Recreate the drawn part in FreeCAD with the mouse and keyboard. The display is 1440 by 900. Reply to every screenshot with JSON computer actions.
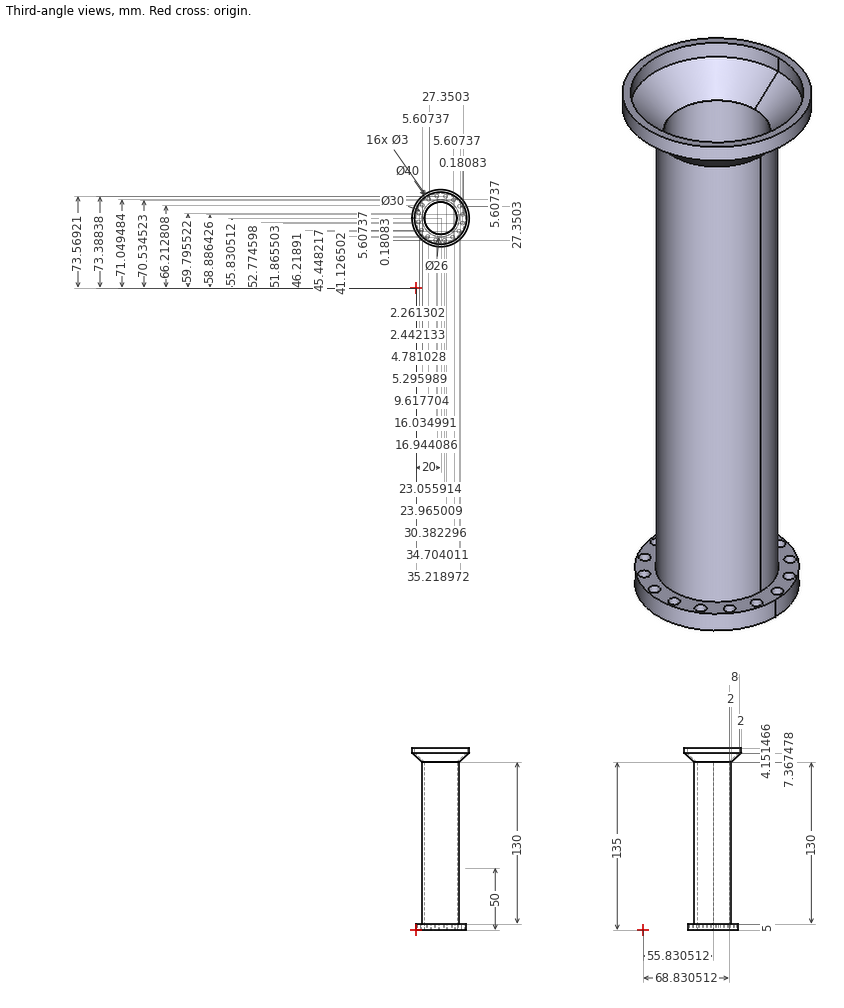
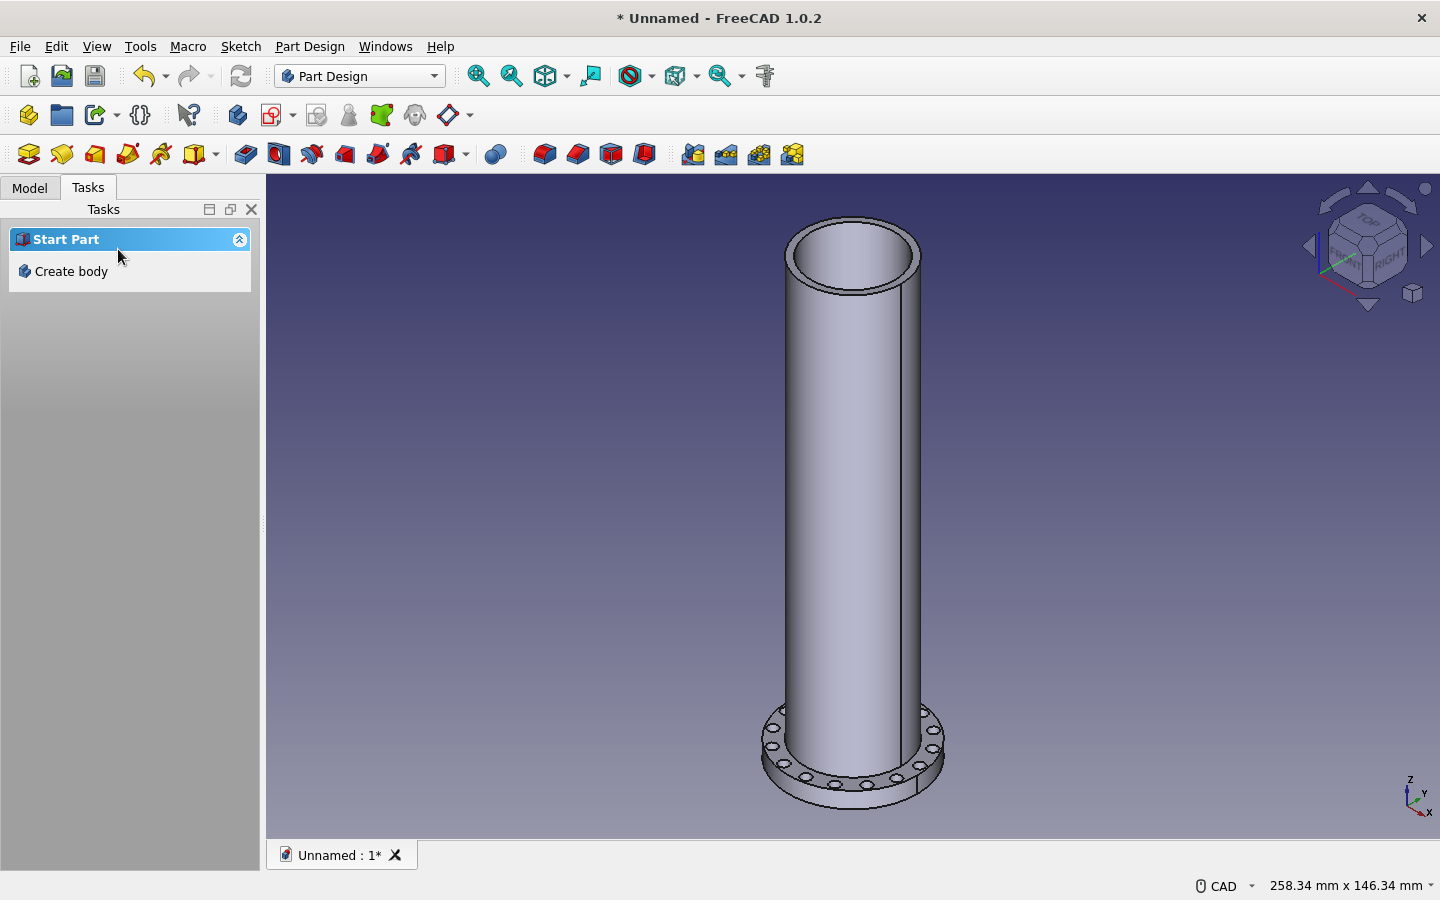
{"action": "left_click", "coordinate": [238, 116]}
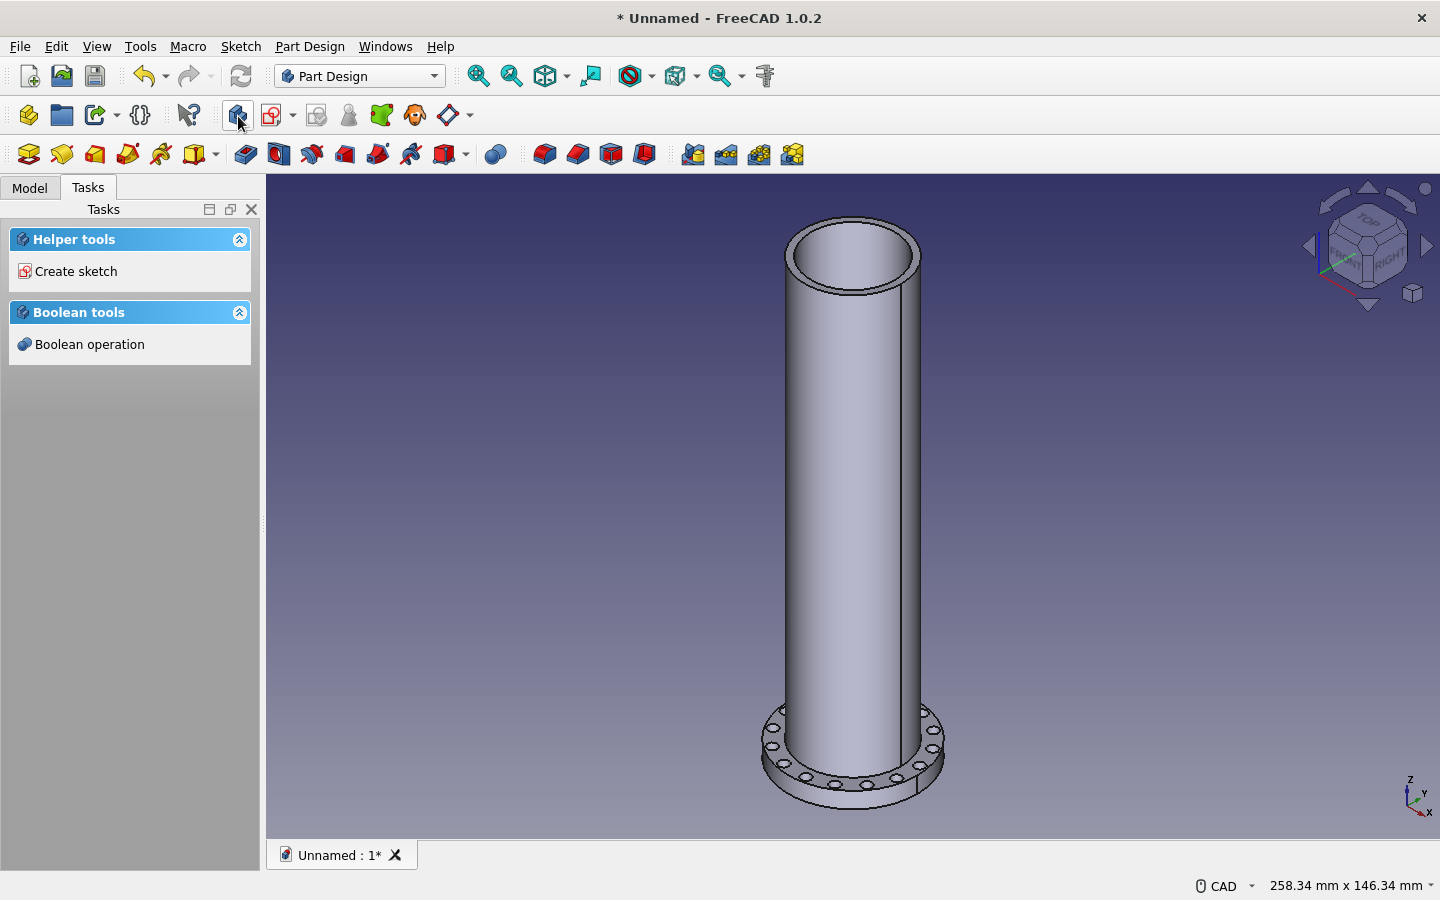
{"action": "left_click", "coordinate": [30, 188]}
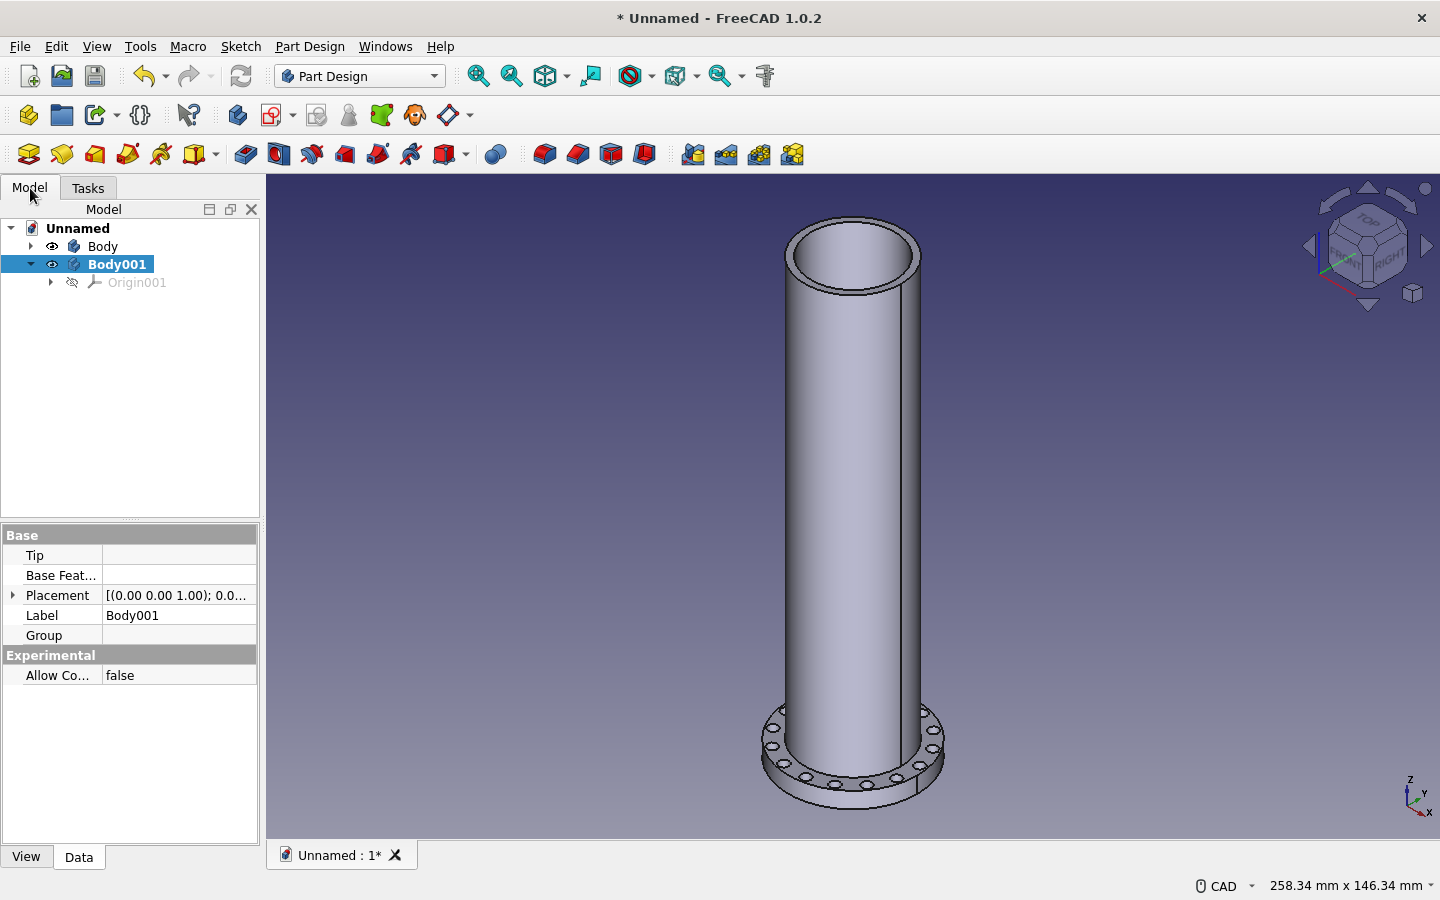
{"action": "left_click", "coordinate": [51, 282]}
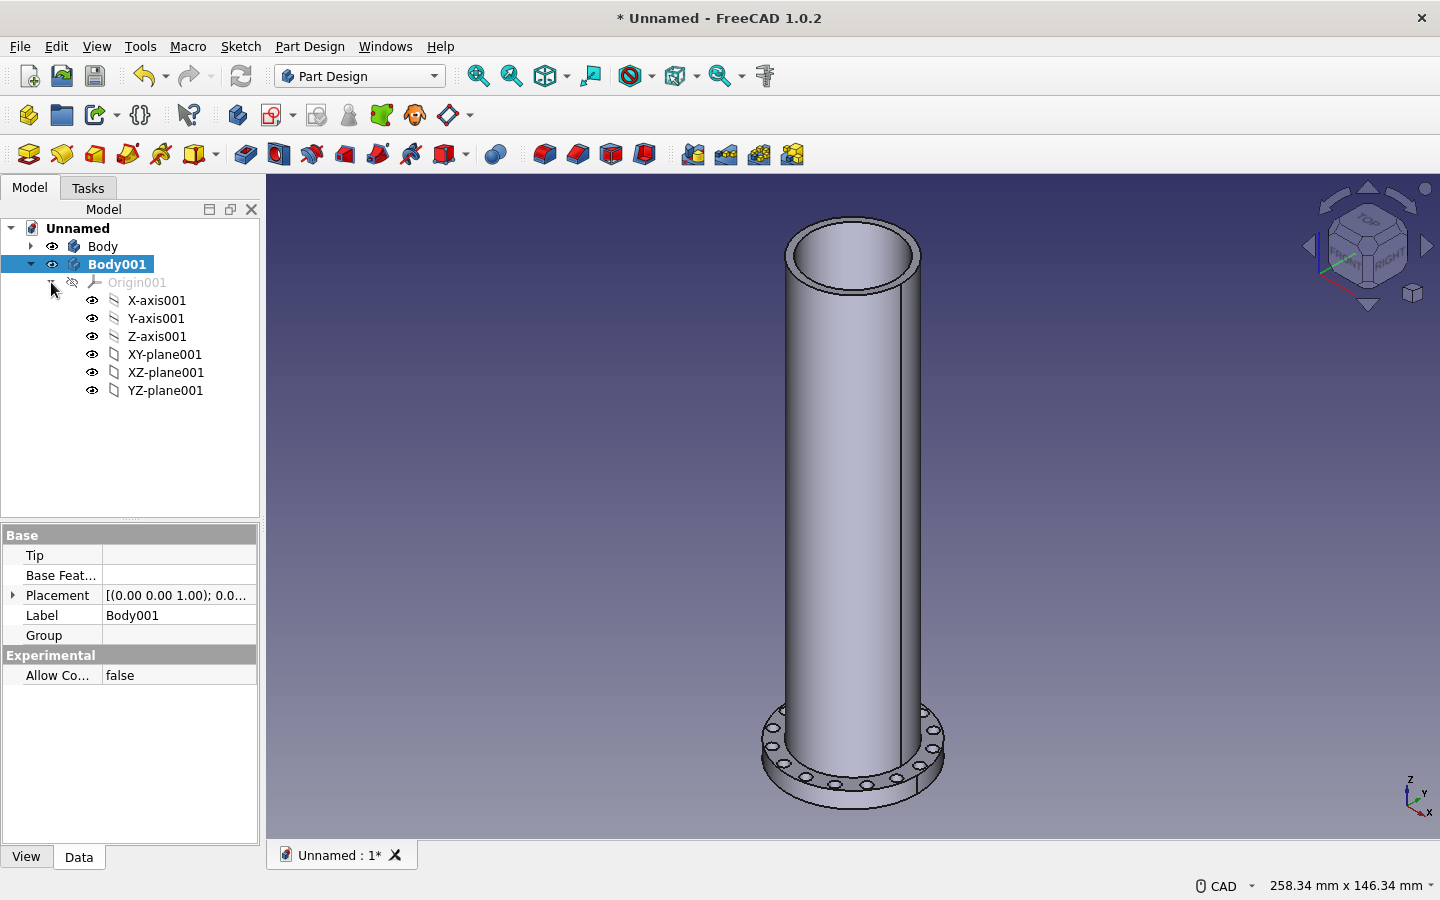
{"action": "left_click", "coordinate": [137, 390]}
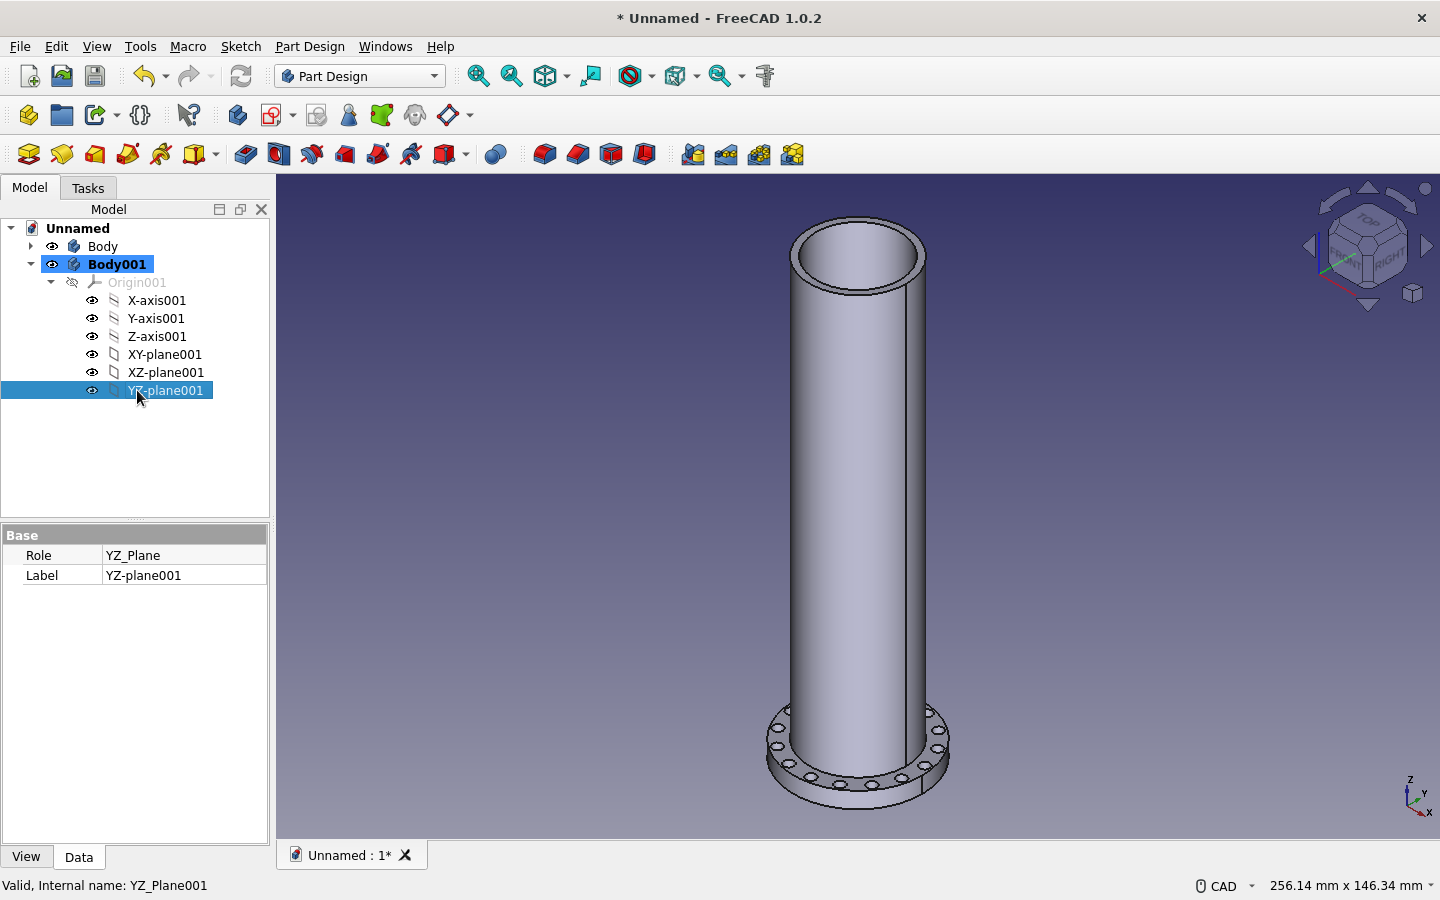
{"action": "left_click", "coordinate": [448, 116]}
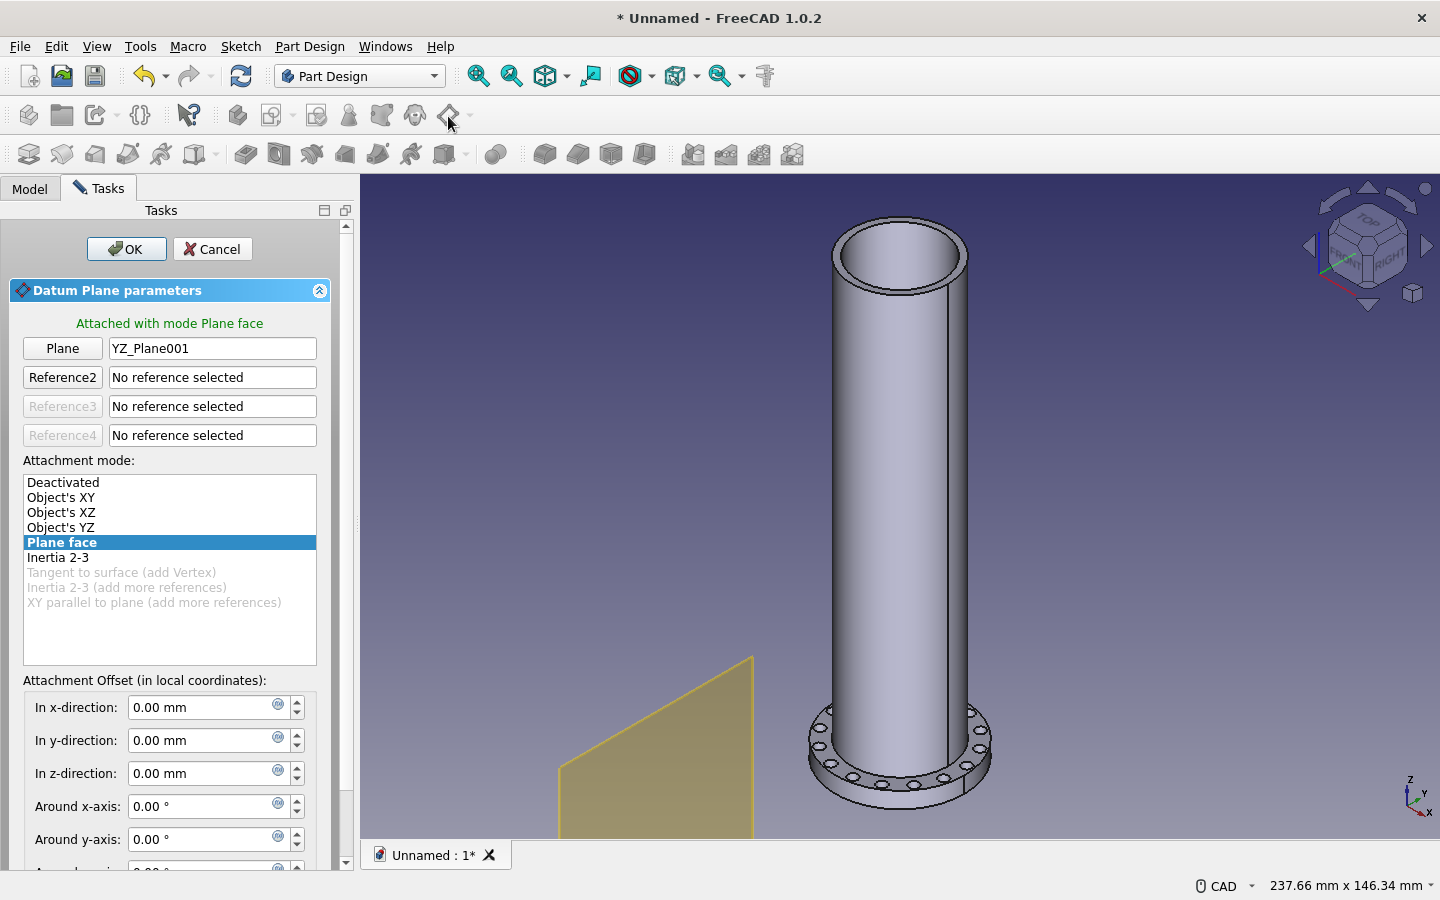
{"action": "triple_click", "coordinate": [210, 774]}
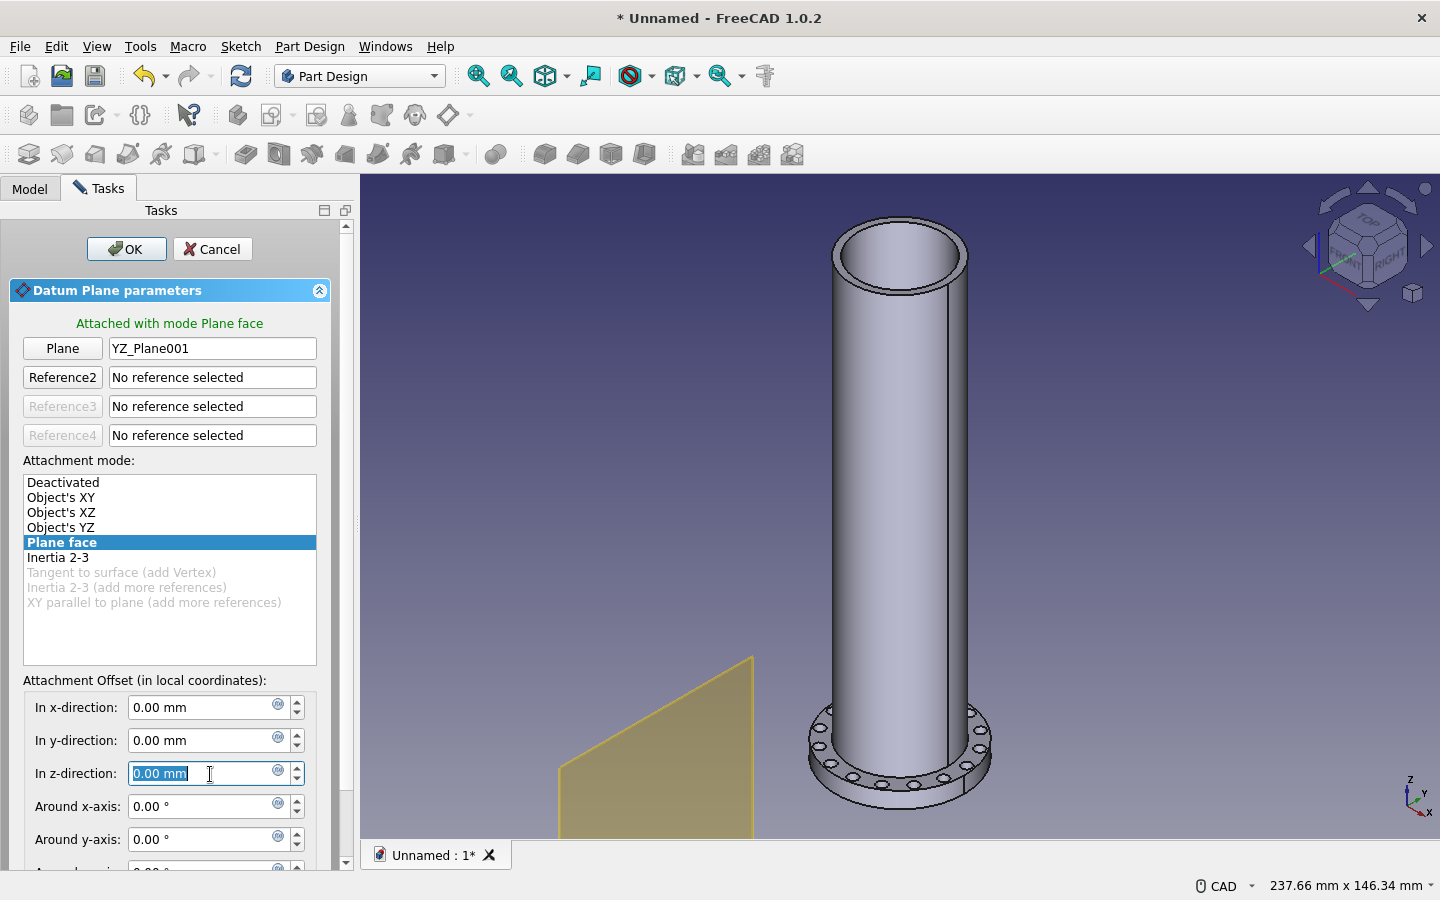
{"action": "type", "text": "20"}
{"action": "key", "text": "Tab"}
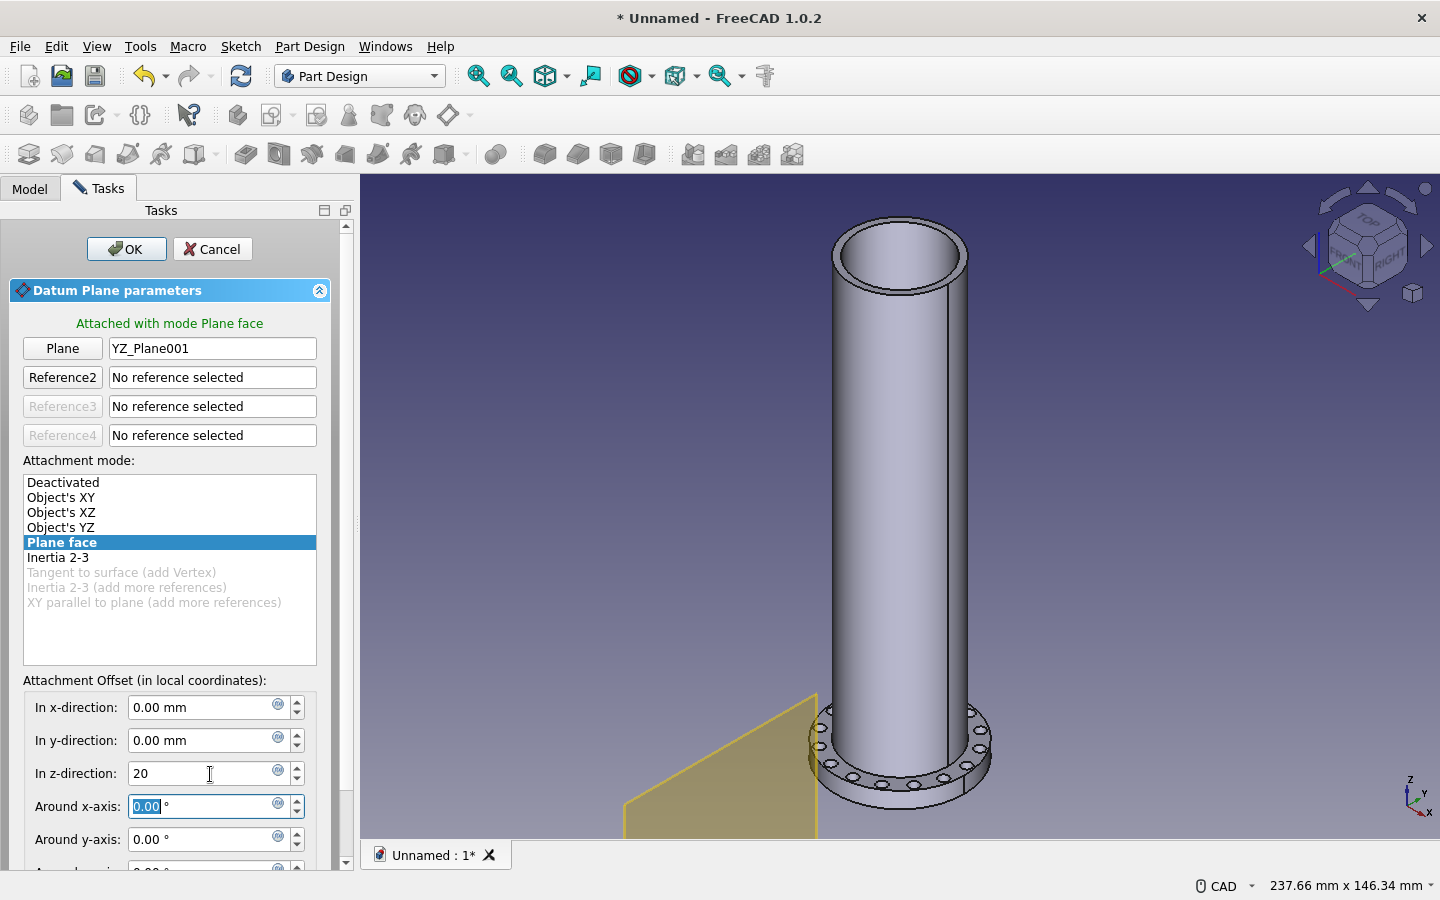
{"action": "left_click", "coordinate": [127, 249]}